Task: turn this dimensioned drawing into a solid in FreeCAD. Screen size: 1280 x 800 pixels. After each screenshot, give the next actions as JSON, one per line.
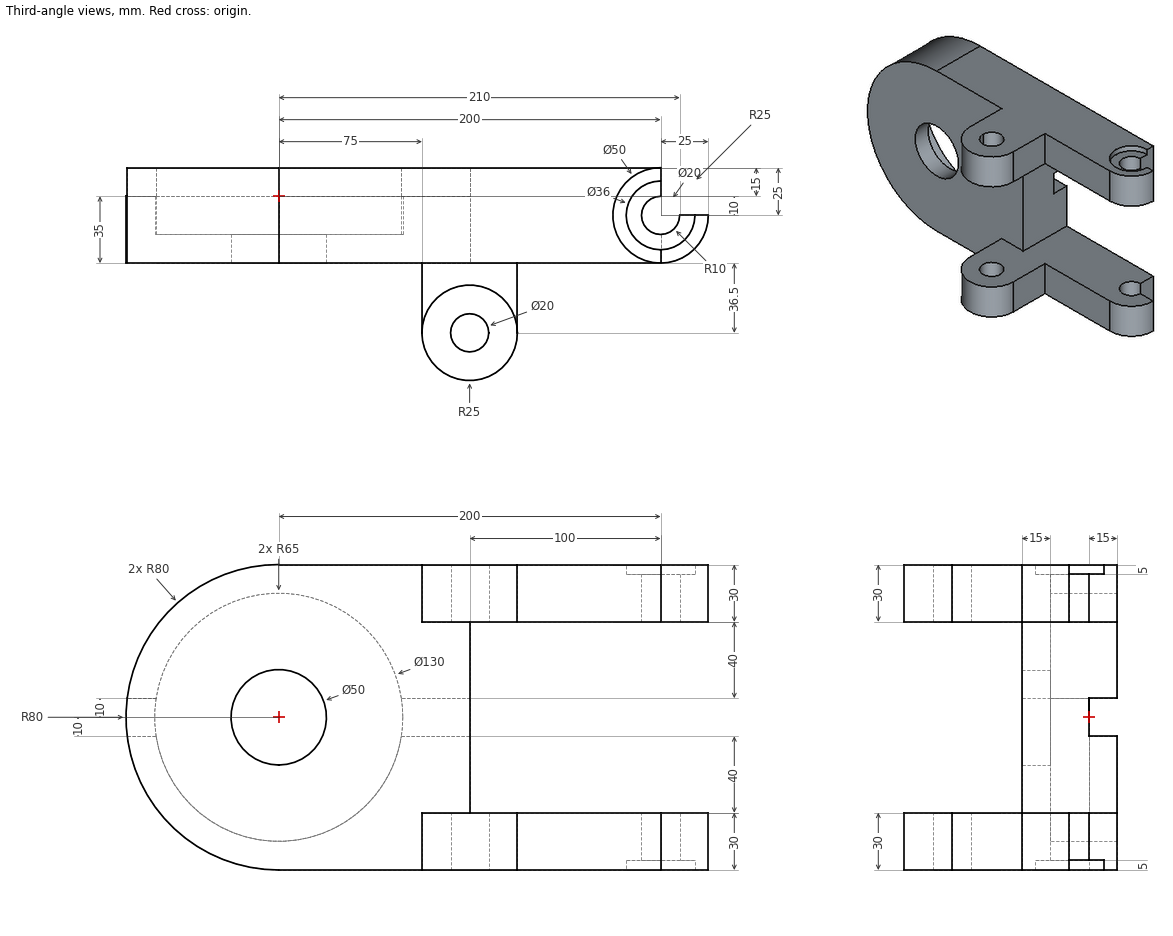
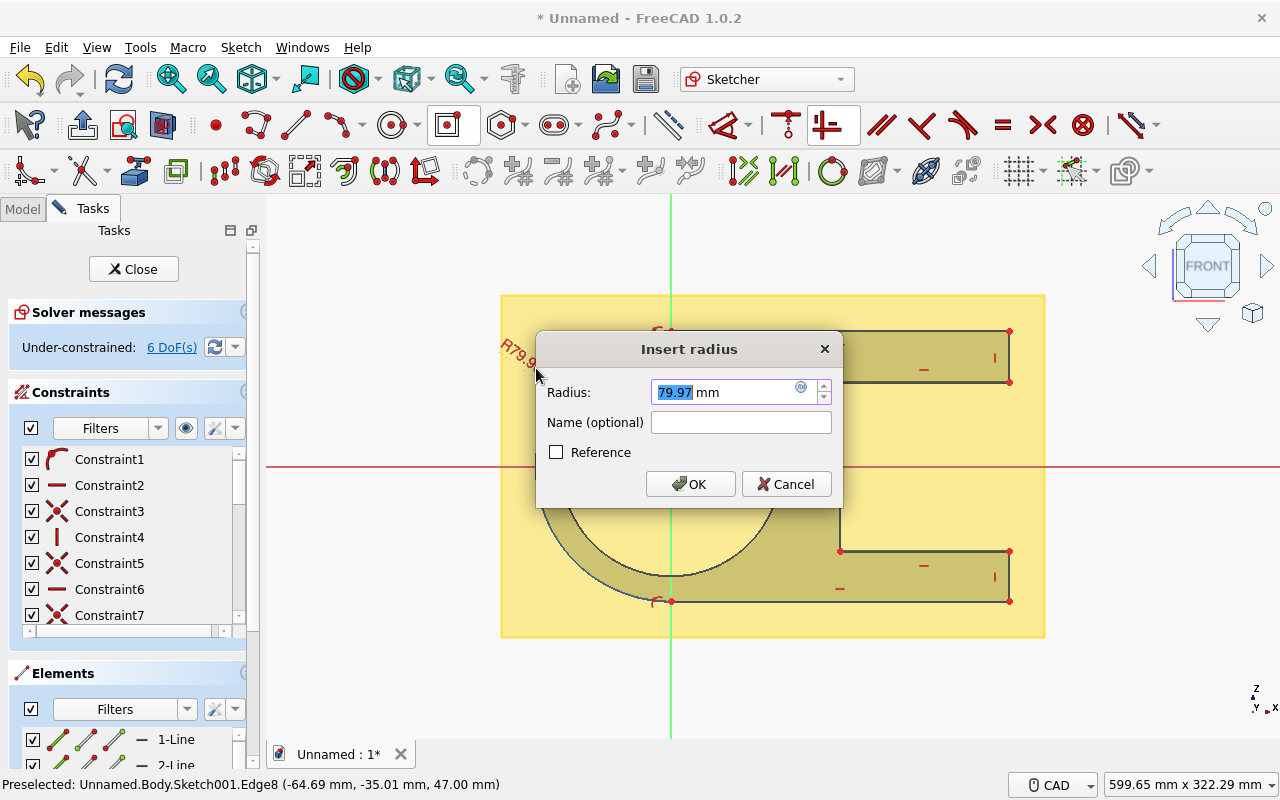
{"action": "type", "text": "80"}
{"action": "key", "text": "Return"}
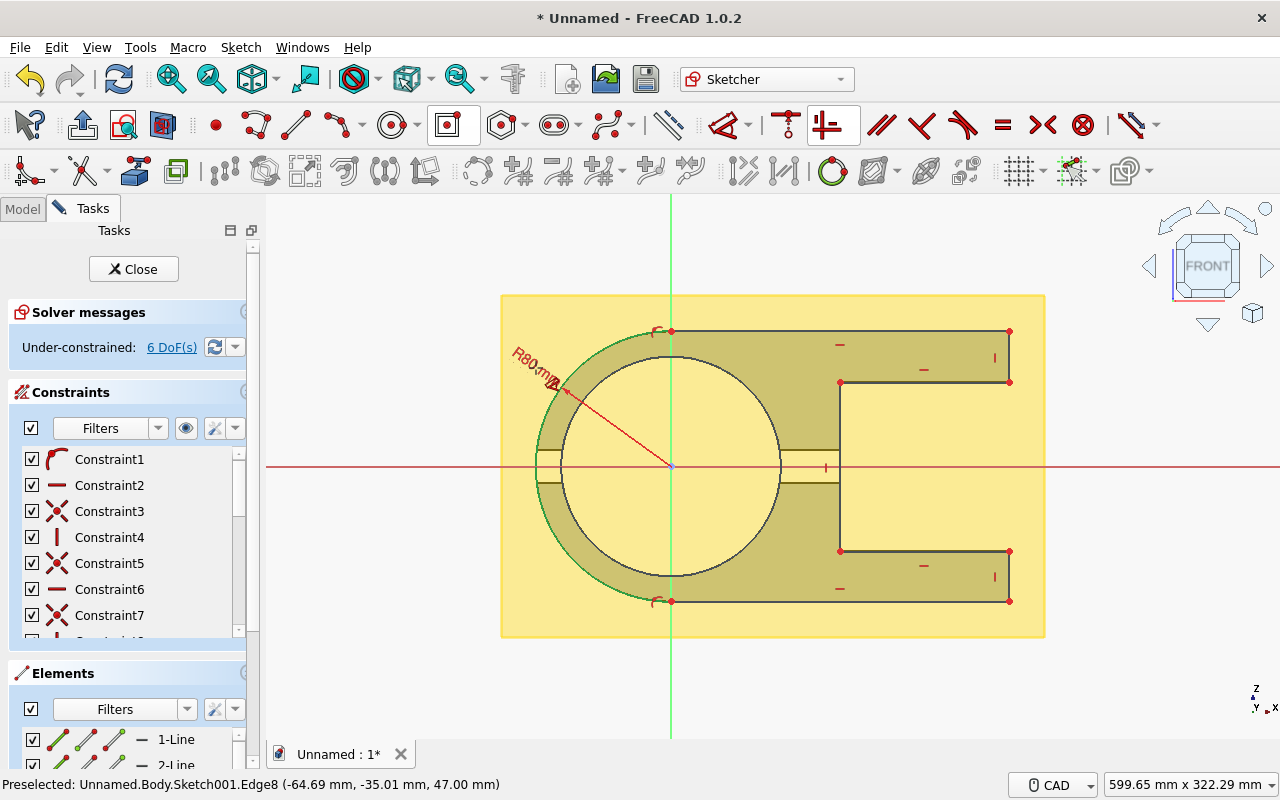
{"action": "left_click", "coordinate": [749, 389]}
{"action": "left_click", "coordinate": [772, 366]}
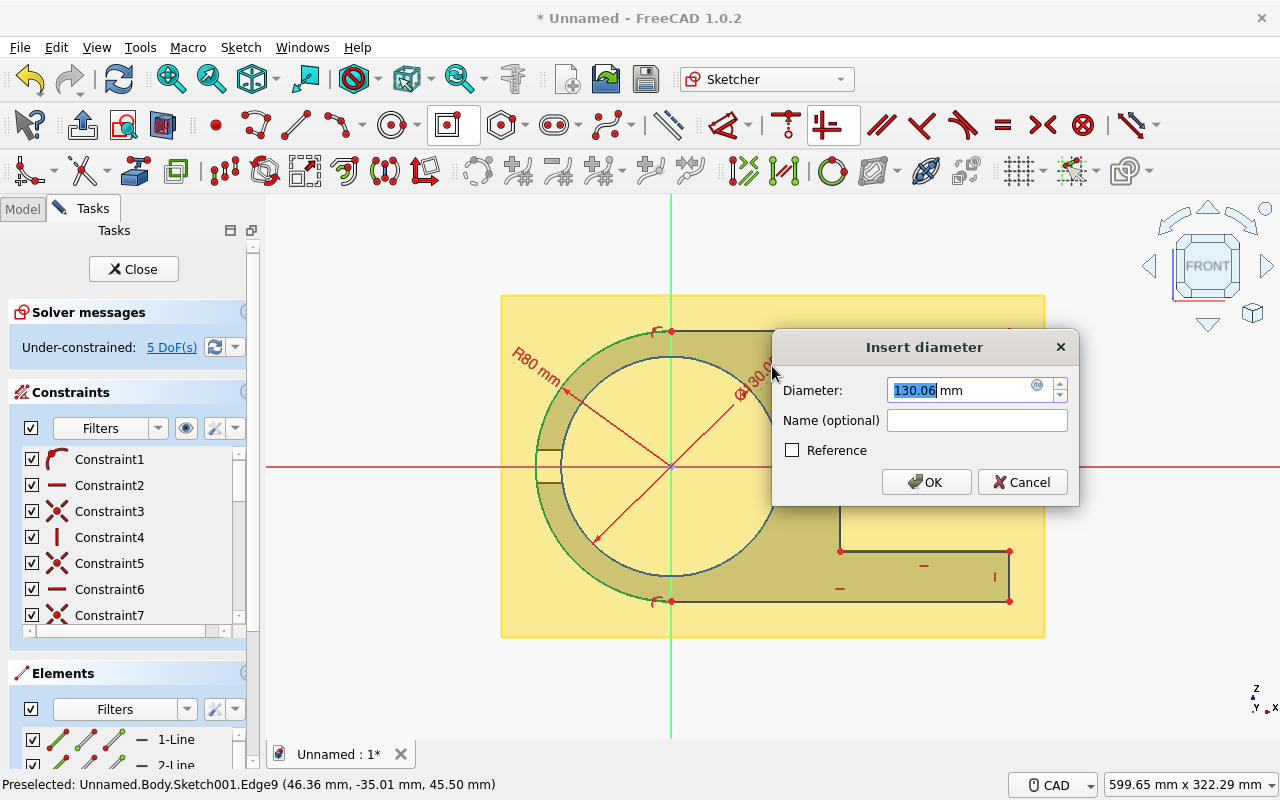
{"action": "type", "text": "130"}
{"action": "key", "text": "Return"}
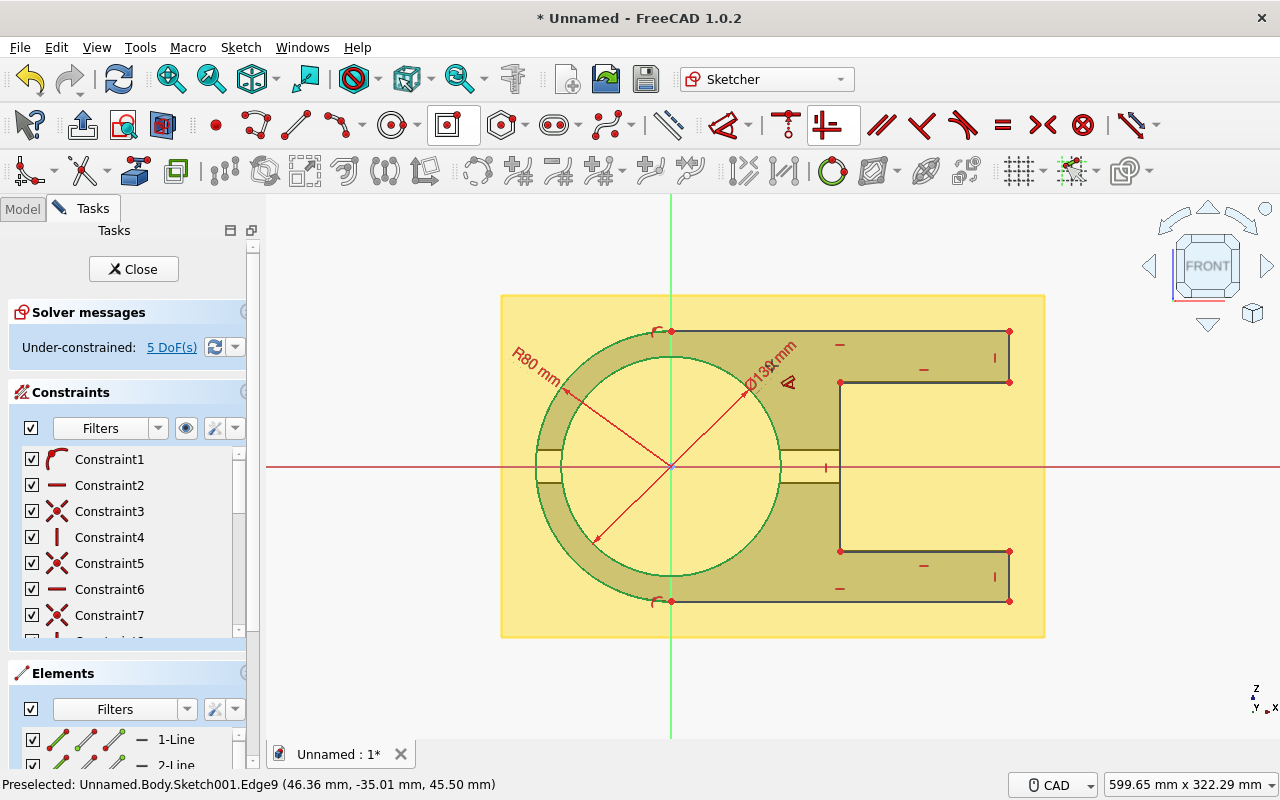
{"action": "left_click", "coordinate": [1009, 587]}
{"action": "left_click", "coordinate": [1043, 577]}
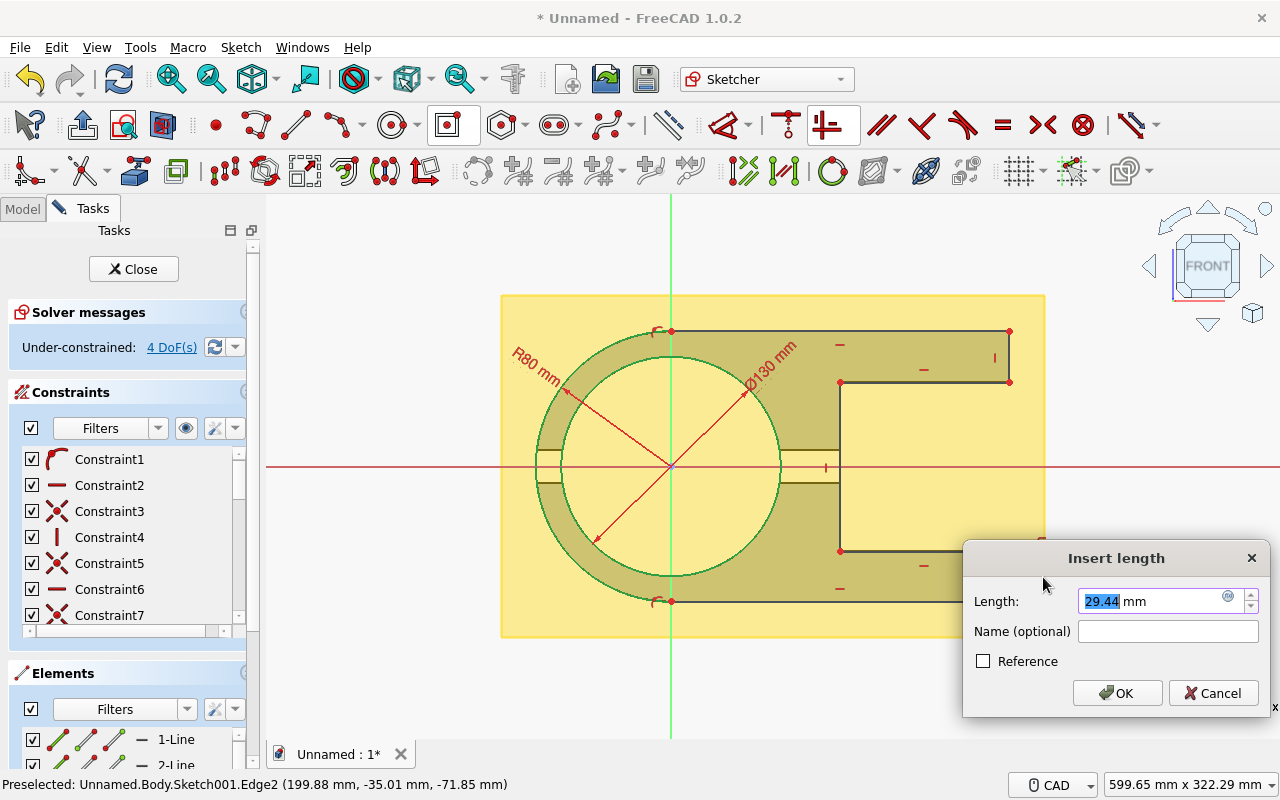
{"action": "type", "text": "30"}
{"action": "key", "text": "Return"}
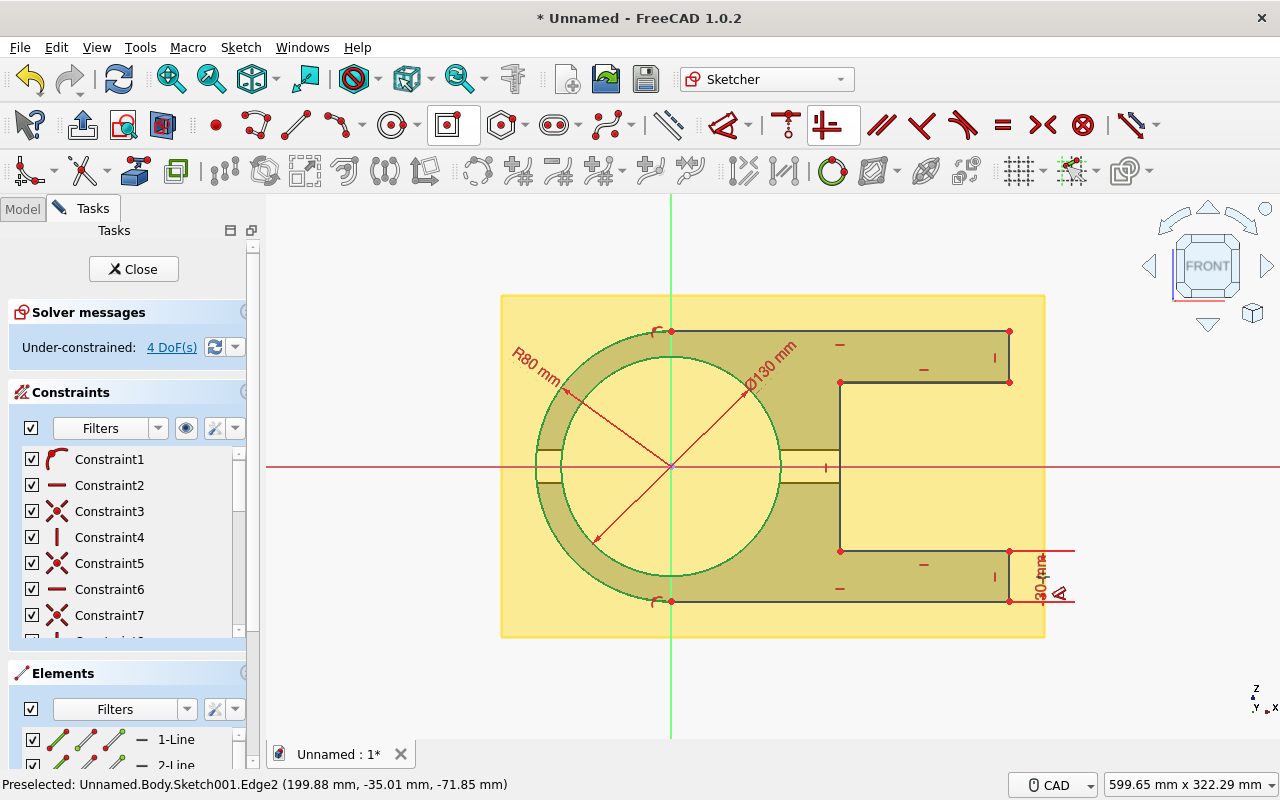
{"action": "left_click", "coordinate": [1009, 367]}
{"action": "left_click", "coordinate": [1043, 357]}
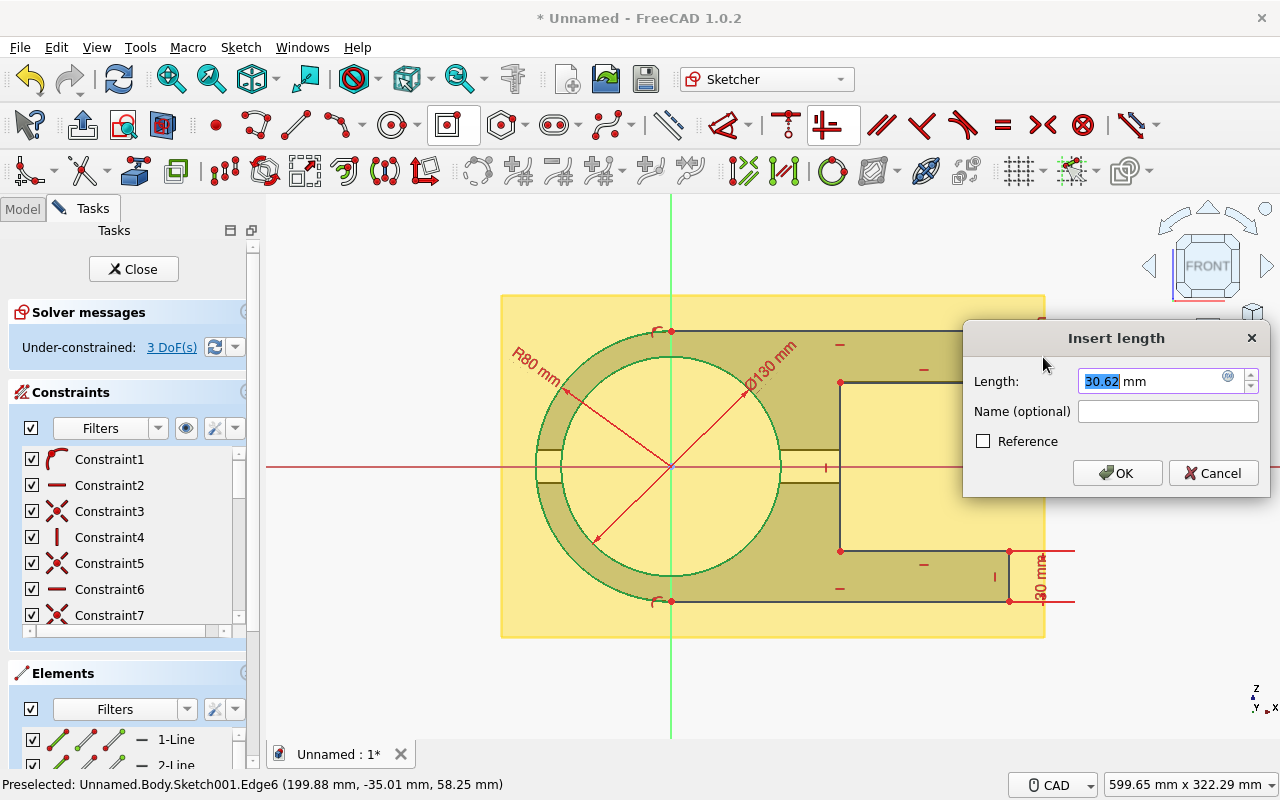
{"action": "type", "text": "30"}
{"action": "key", "text": "Return"}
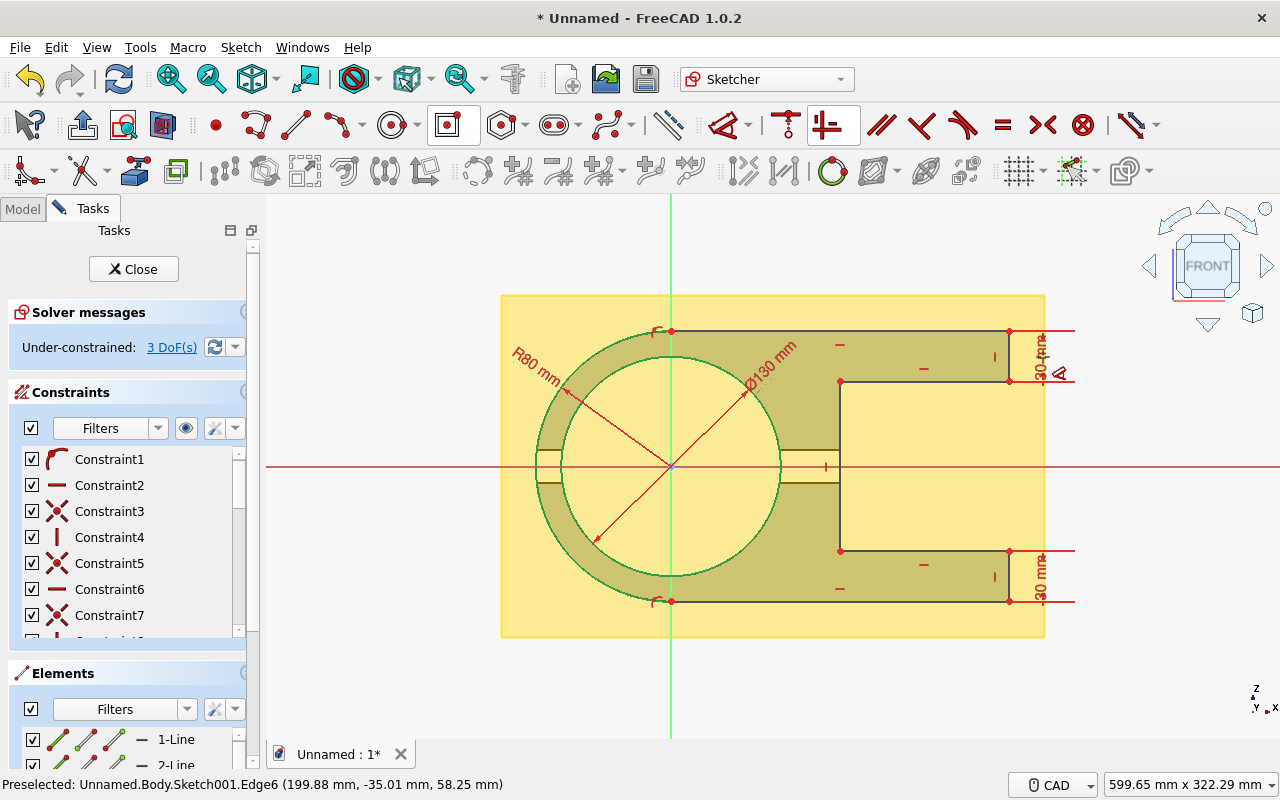
{"action": "left_click", "coordinate": [772, 602]}
{"action": "left_click", "coordinate": [840, 636]}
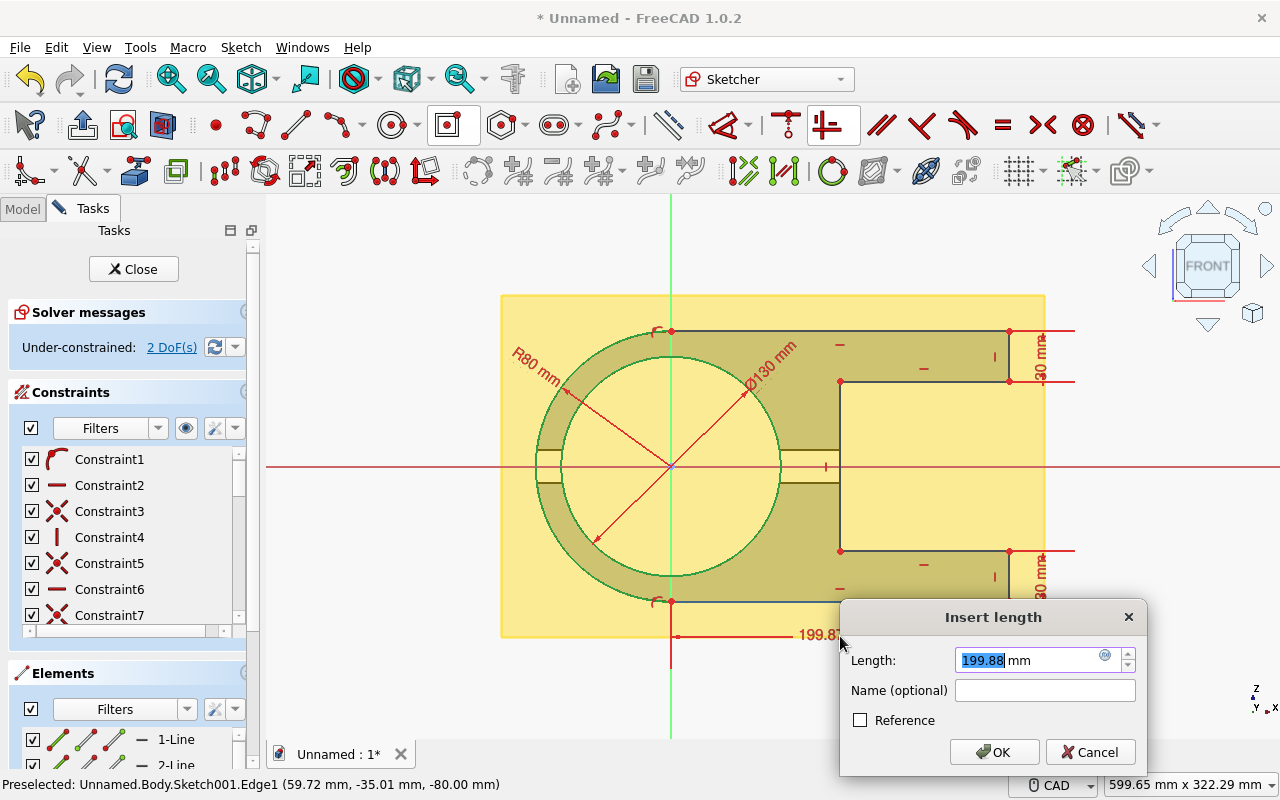
{"action": "type", "text": "200"}
{"action": "key", "text": "Return"}